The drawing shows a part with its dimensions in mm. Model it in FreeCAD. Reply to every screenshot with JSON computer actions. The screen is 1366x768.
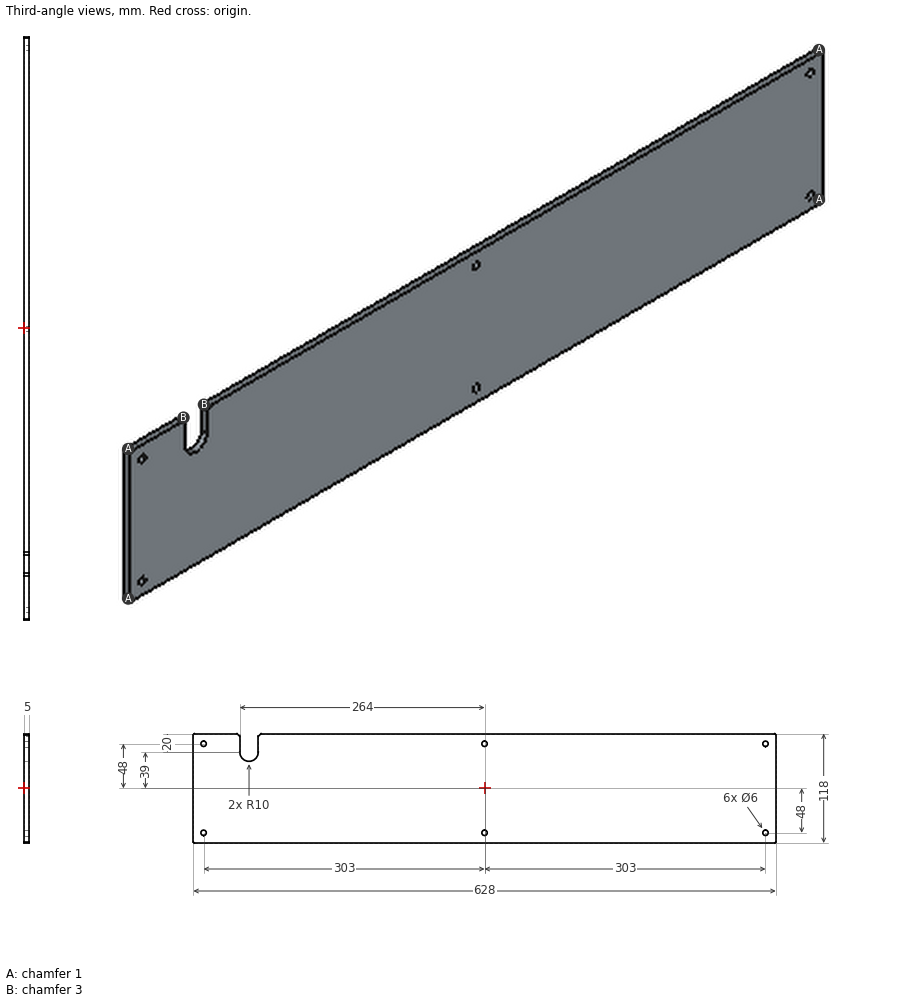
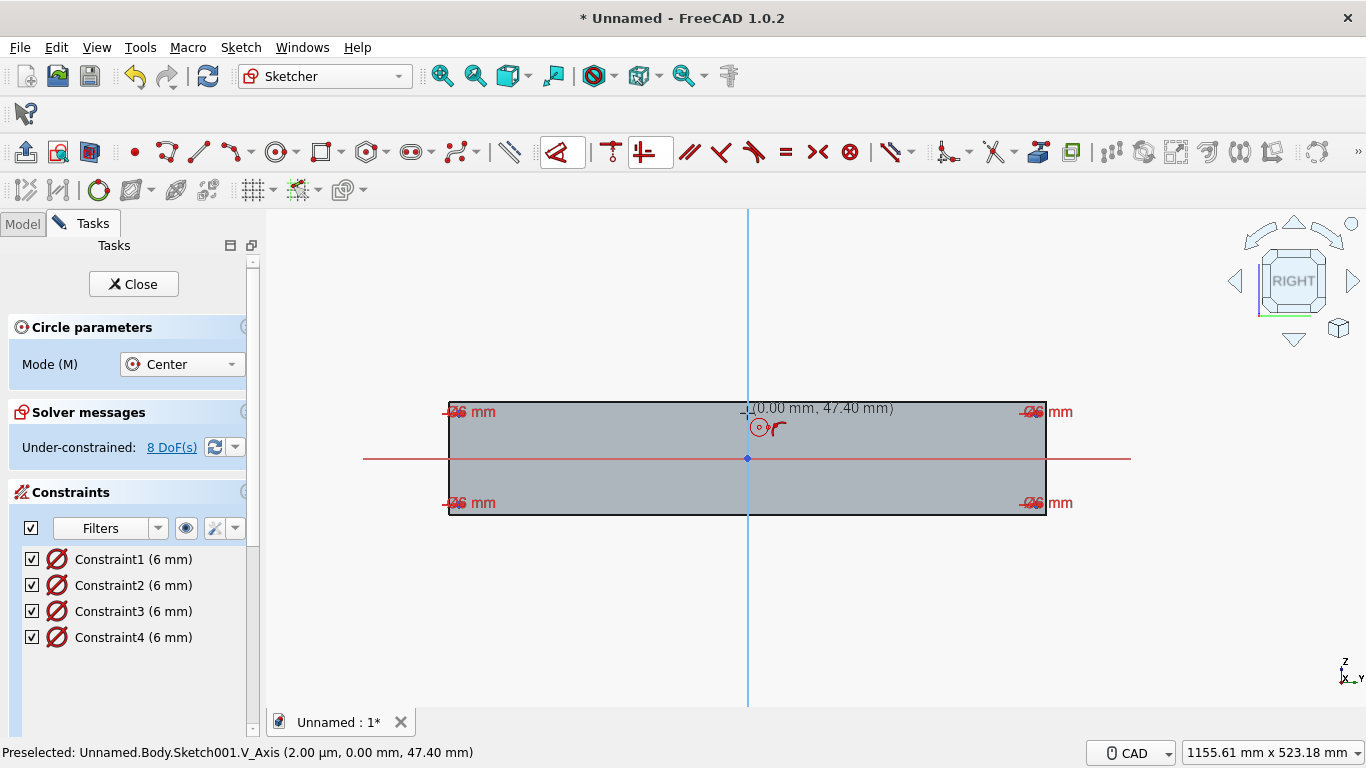
{"action": "left_click", "coordinate": [748, 413]}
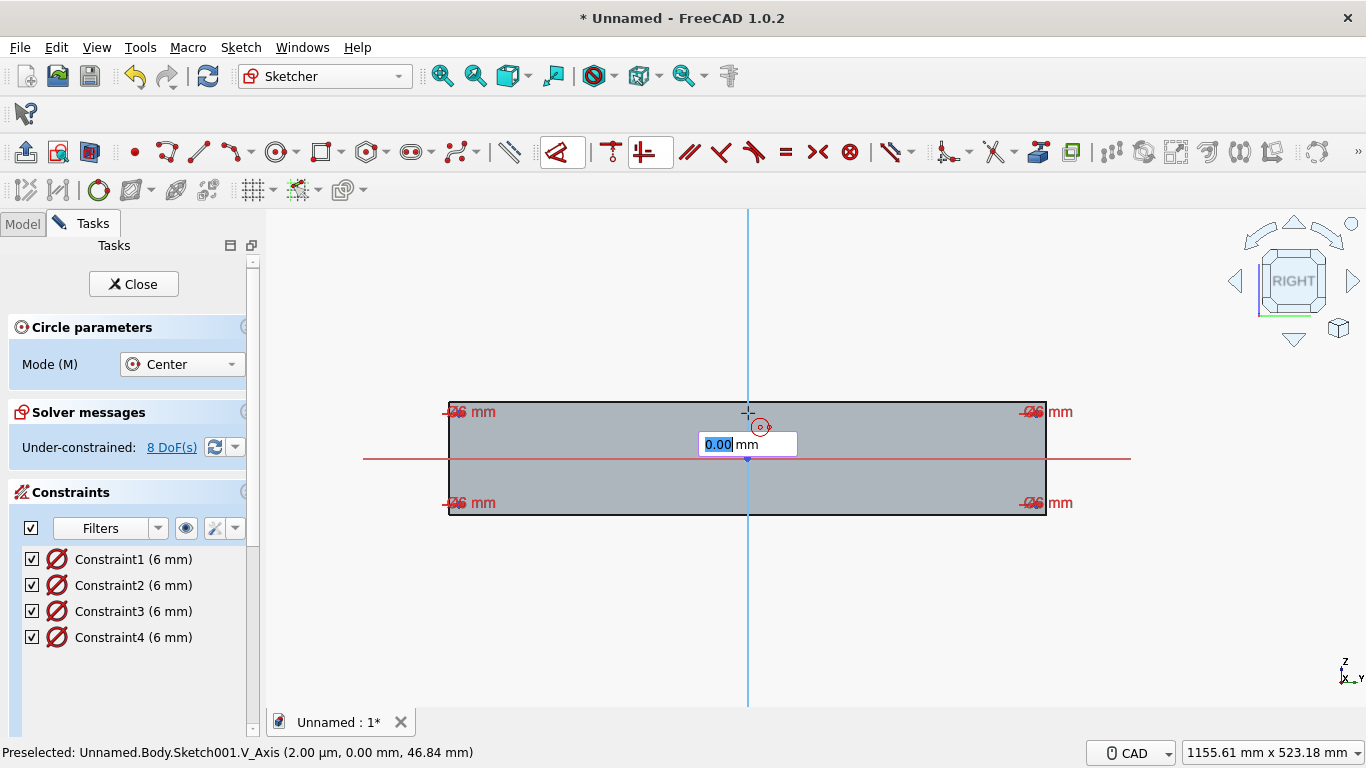
{"action": "scroll", "coordinate": [750, 412], "scroll_direction": "up", "scroll_amount": 9}
{"action": "mouse_move", "coordinate": [749, 409]}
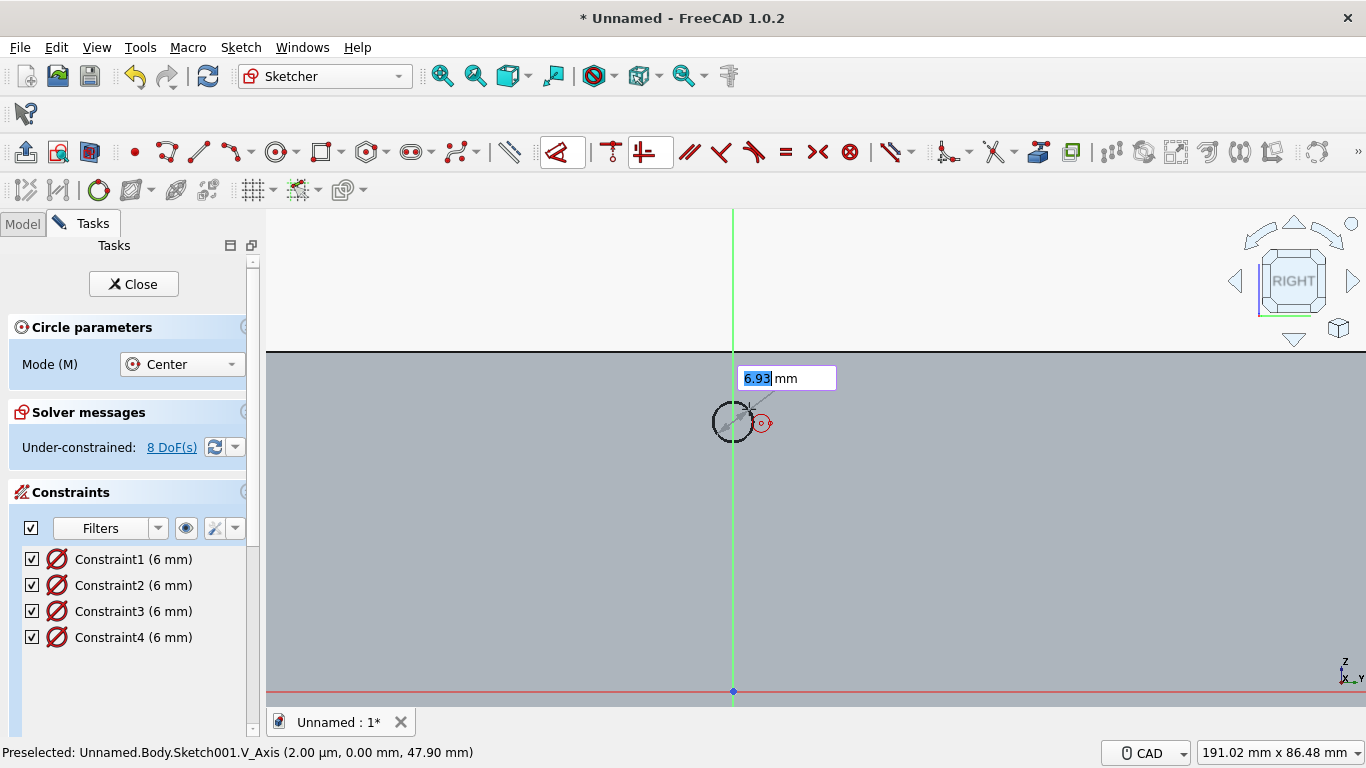
{"action": "type", "text": "6"}
{"action": "key", "text": "Return"}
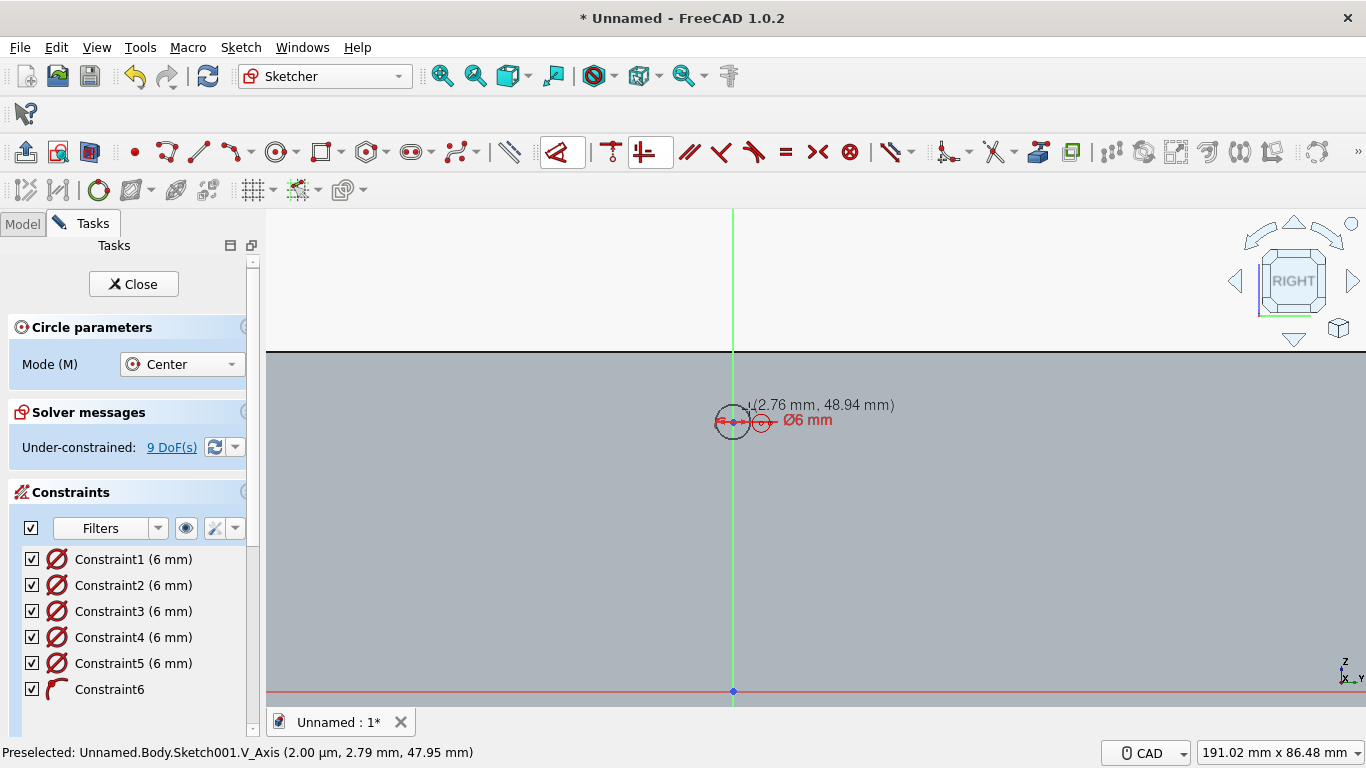
{"action": "scroll", "coordinate": [750, 412], "scroll_direction": "down", "scroll_amount": 9}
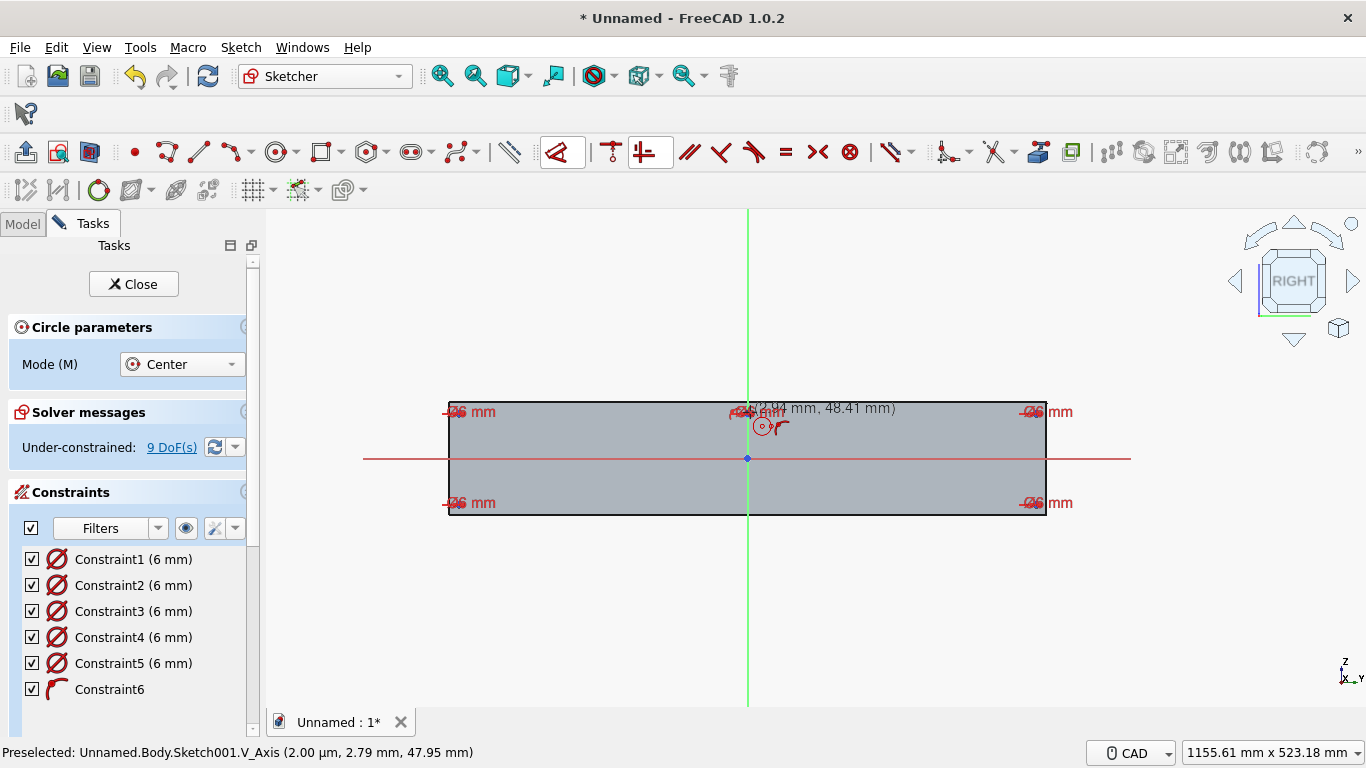
{"action": "scroll", "coordinate": [748, 504], "scroll_direction": "up", "scroll_amount": 11}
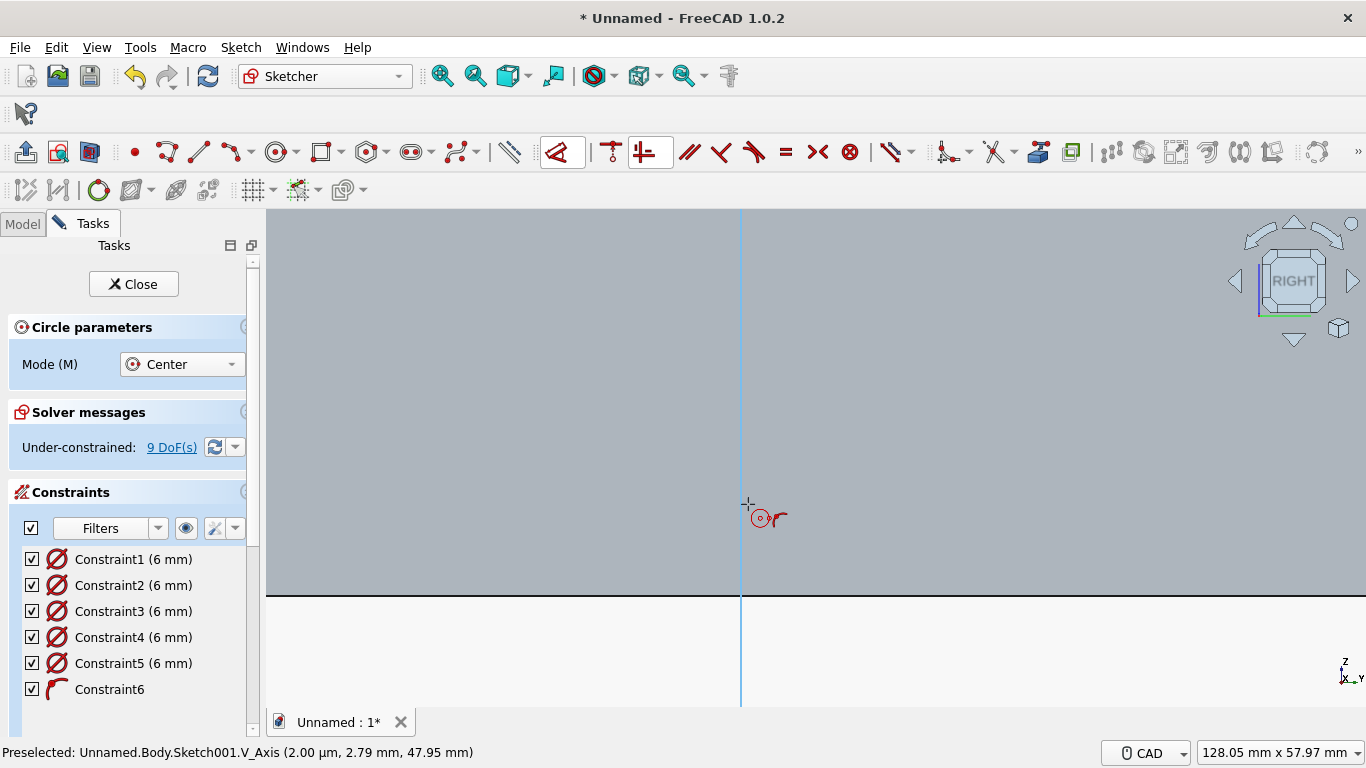
{"action": "scroll", "coordinate": [748, 504], "scroll_direction": "down", "scroll_amount": 11}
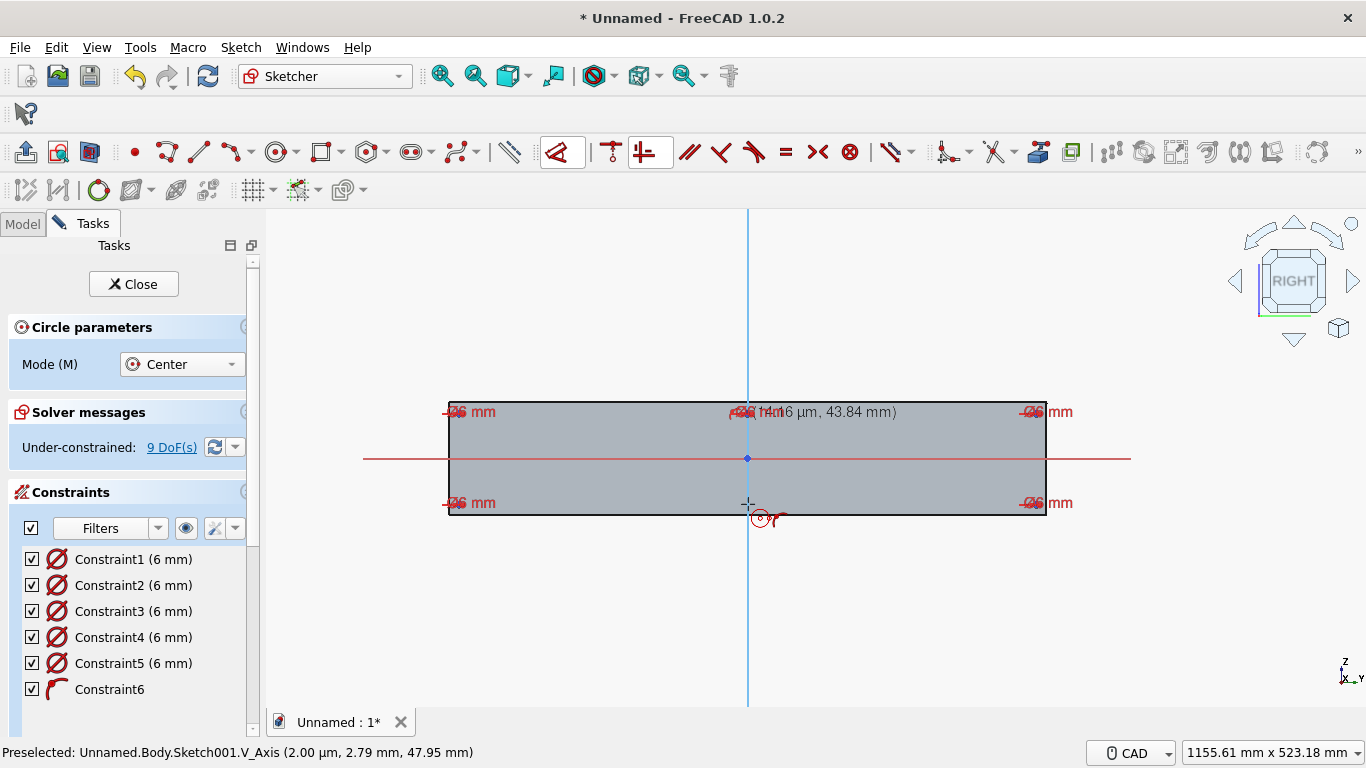
{"action": "left_click", "coordinate": [748, 504]}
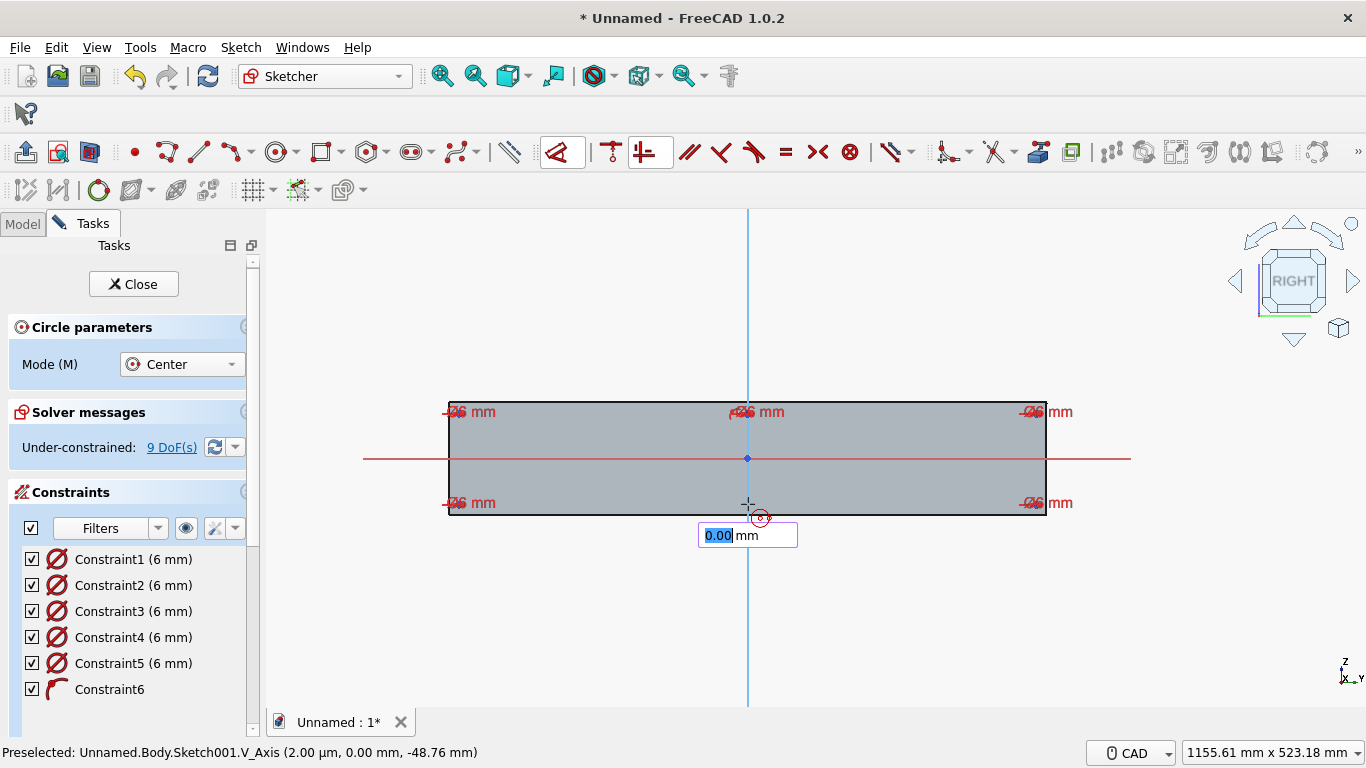
{"action": "scroll", "coordinate": [750, 503], "scroll_direction": "up", "scroll_amount": 9}
{"action": "mouse_move", "coordinate": [749, 502]}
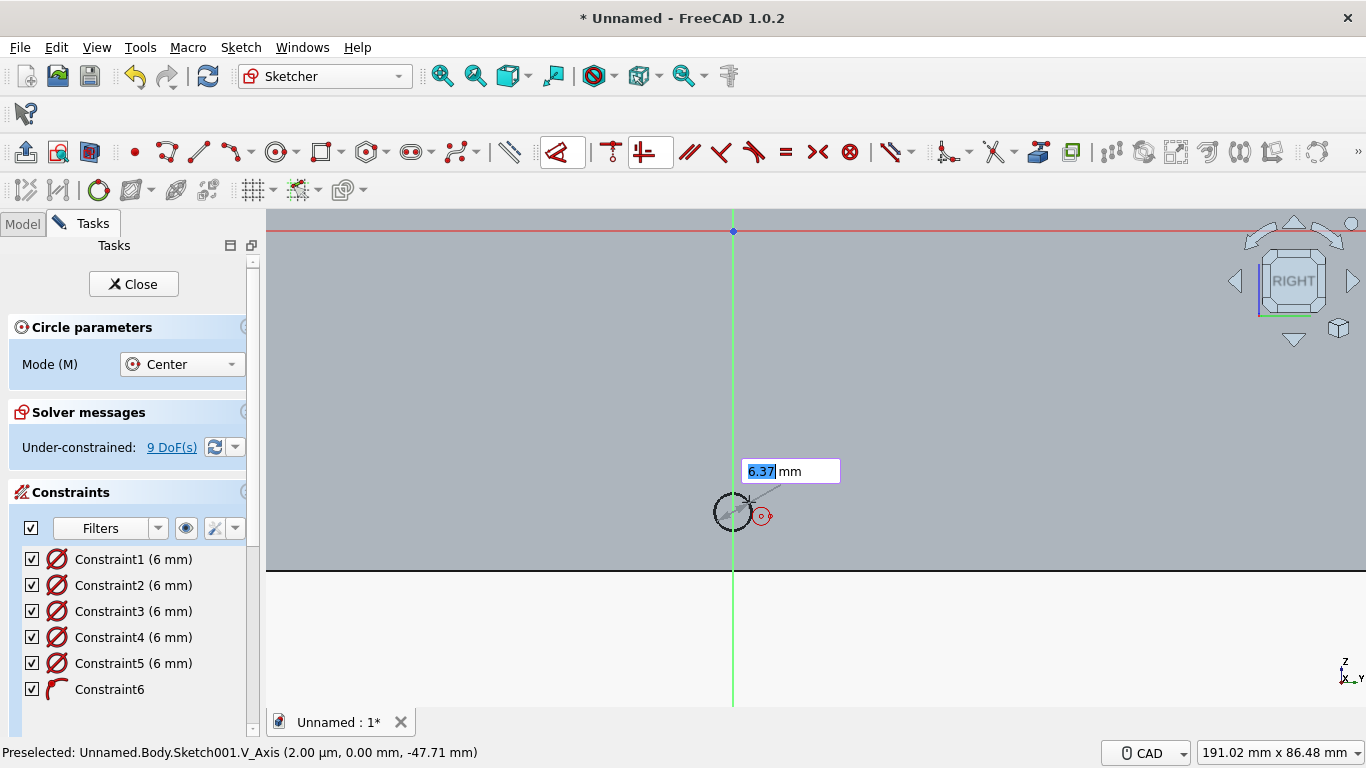
{"action": "type", "text": "6"}
{"action": "key", "text": "Return"}
{"action": "key", "text": "Escape"}